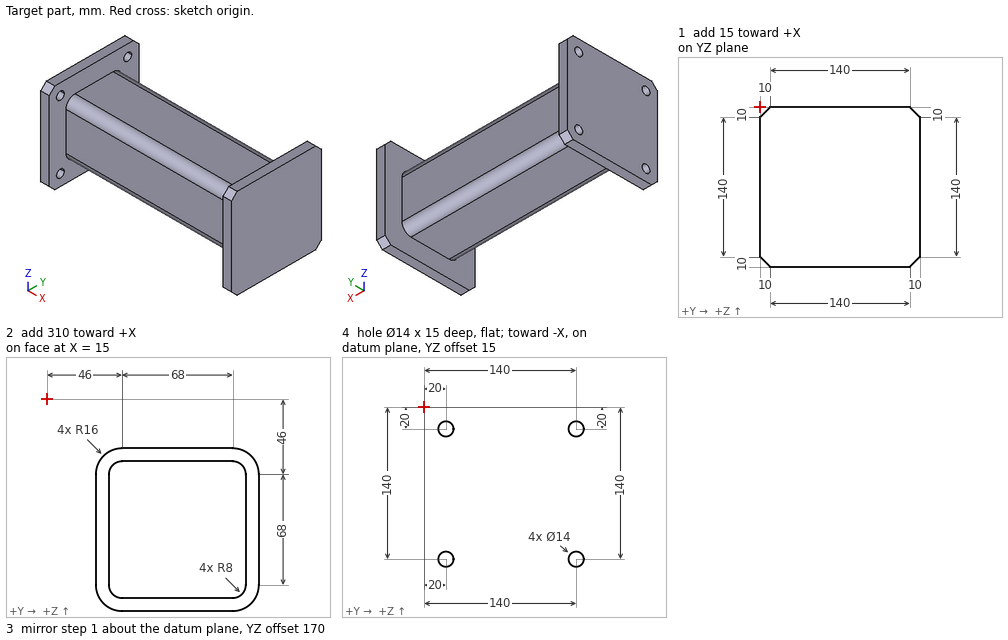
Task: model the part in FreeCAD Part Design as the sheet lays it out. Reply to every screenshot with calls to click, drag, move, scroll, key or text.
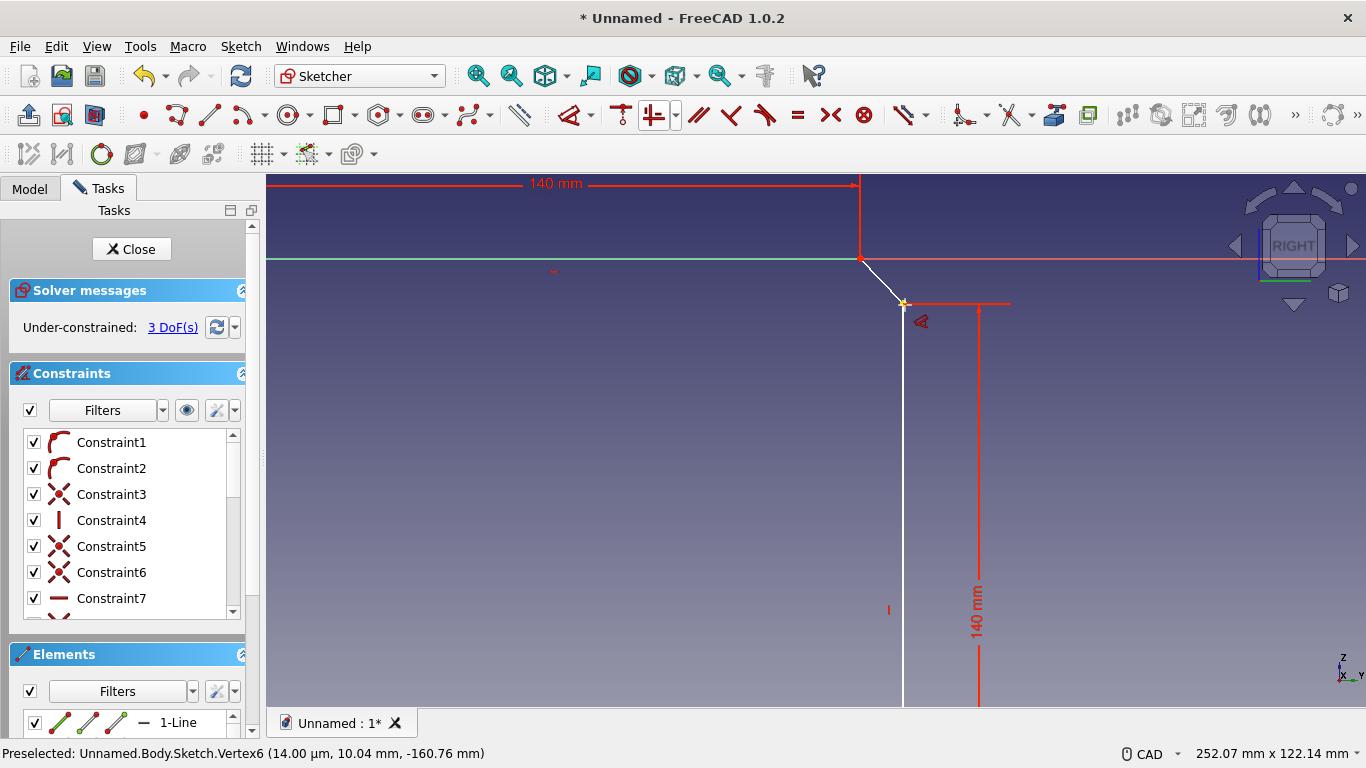
click(903, 304)
click(937, 281)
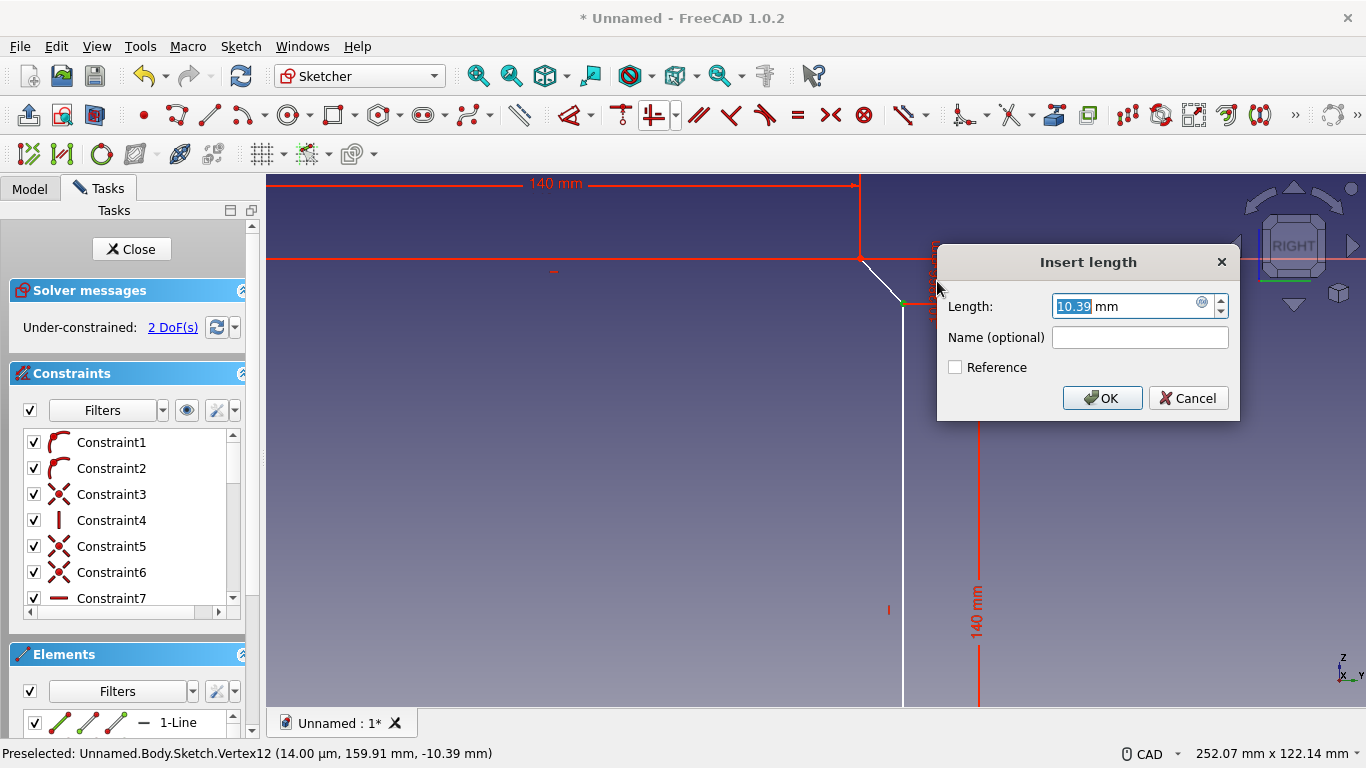
text(10)
key(Return)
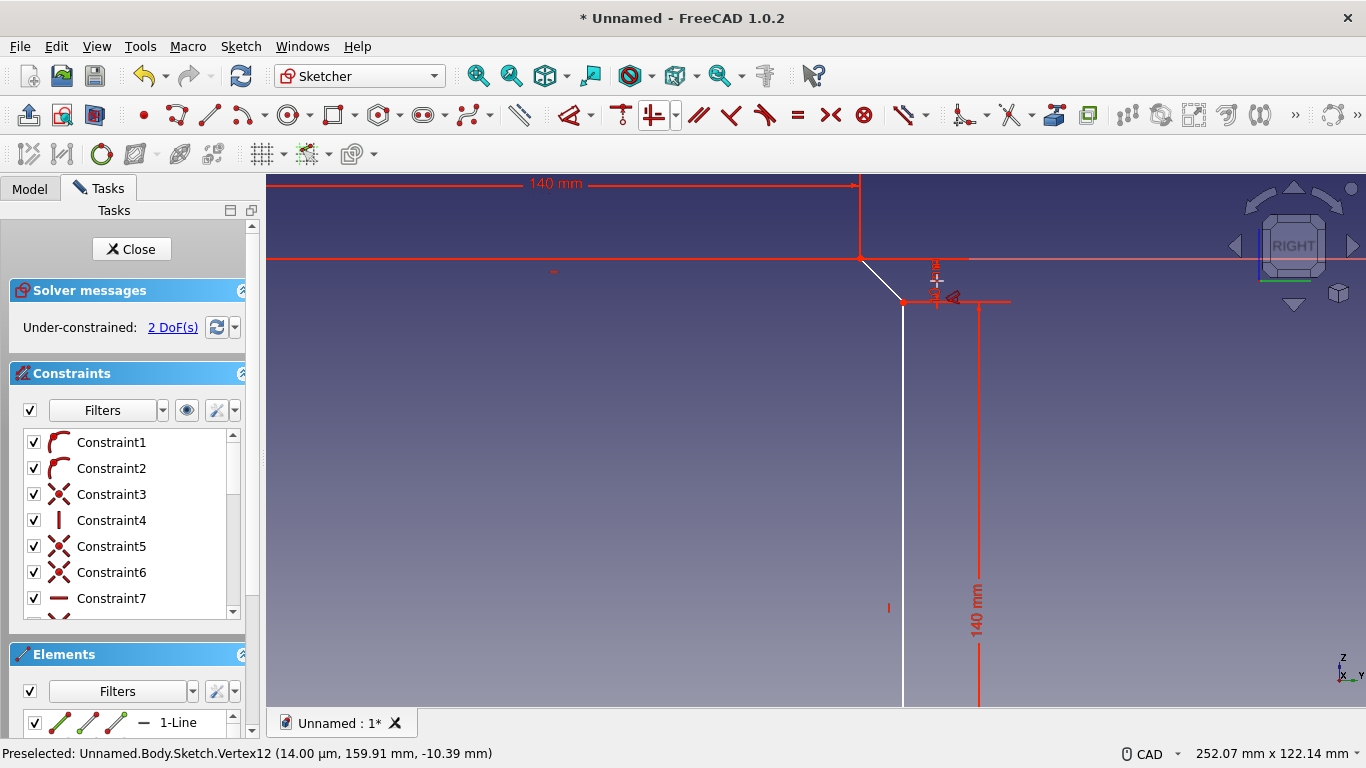
scroll(905, 304, down, 4)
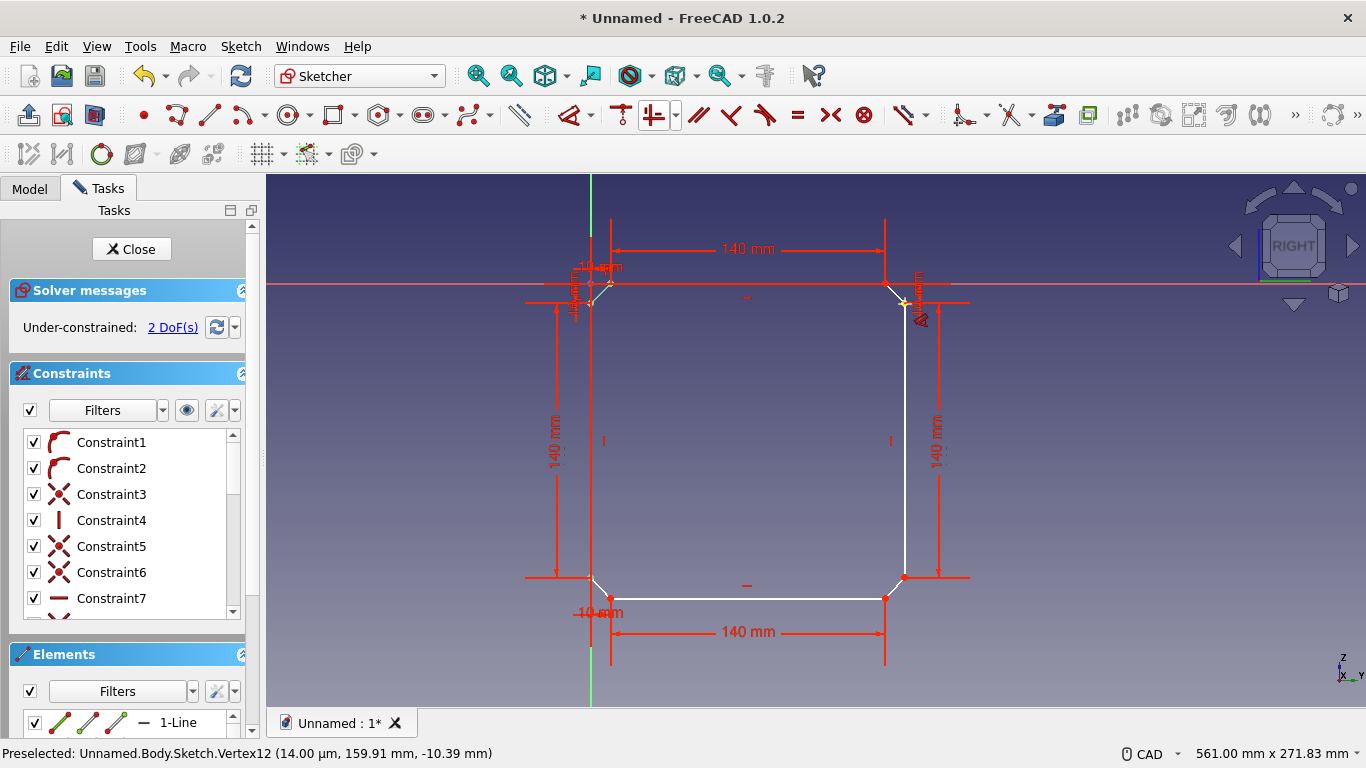
scroll(597, 584, up, 5)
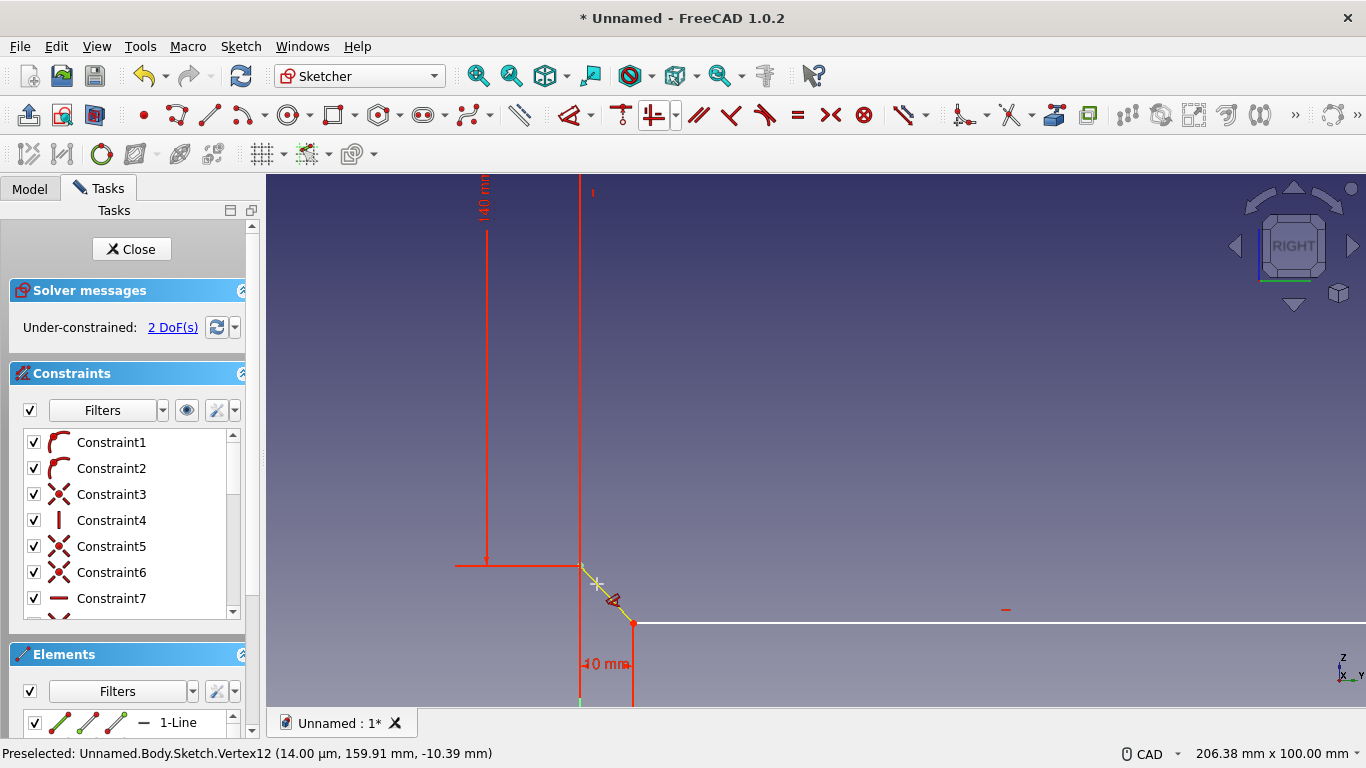
click(596, 583)
click(546, 595)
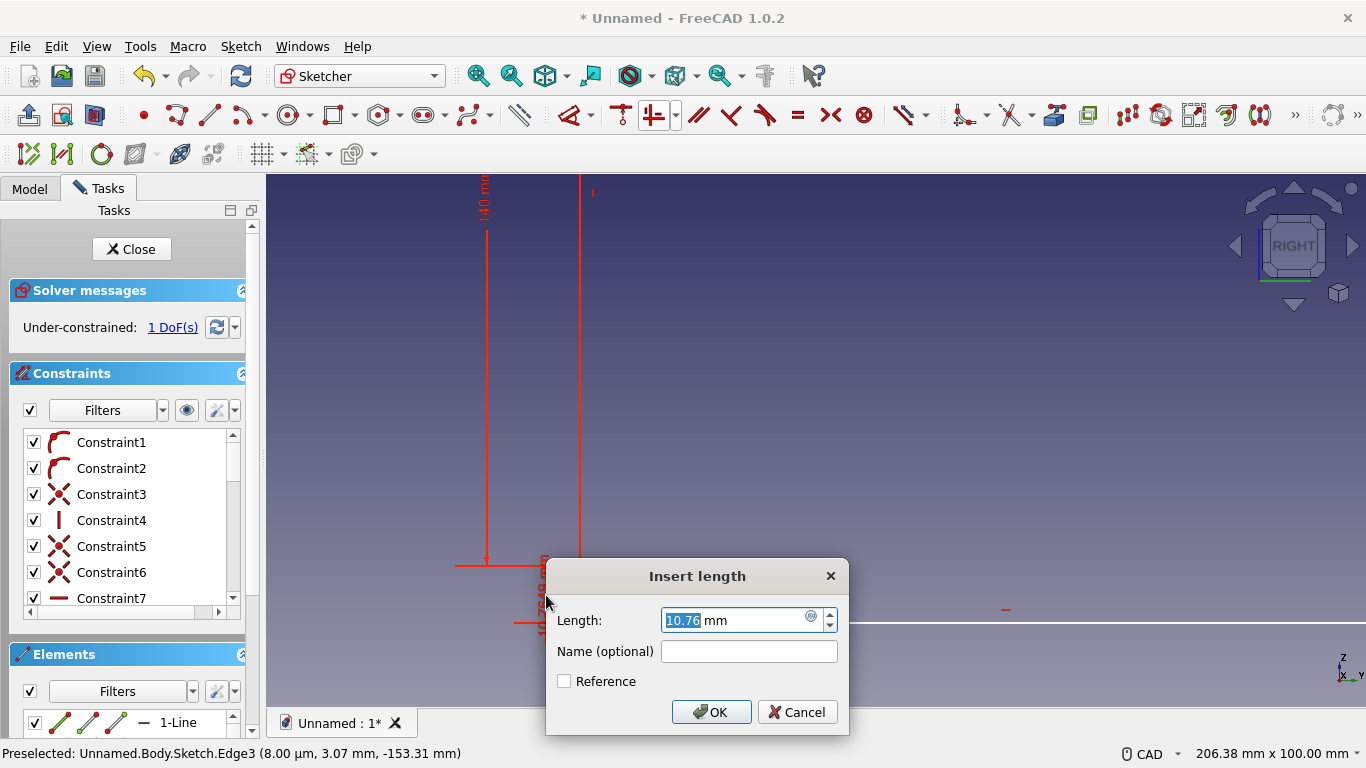
text(10)
key(Return)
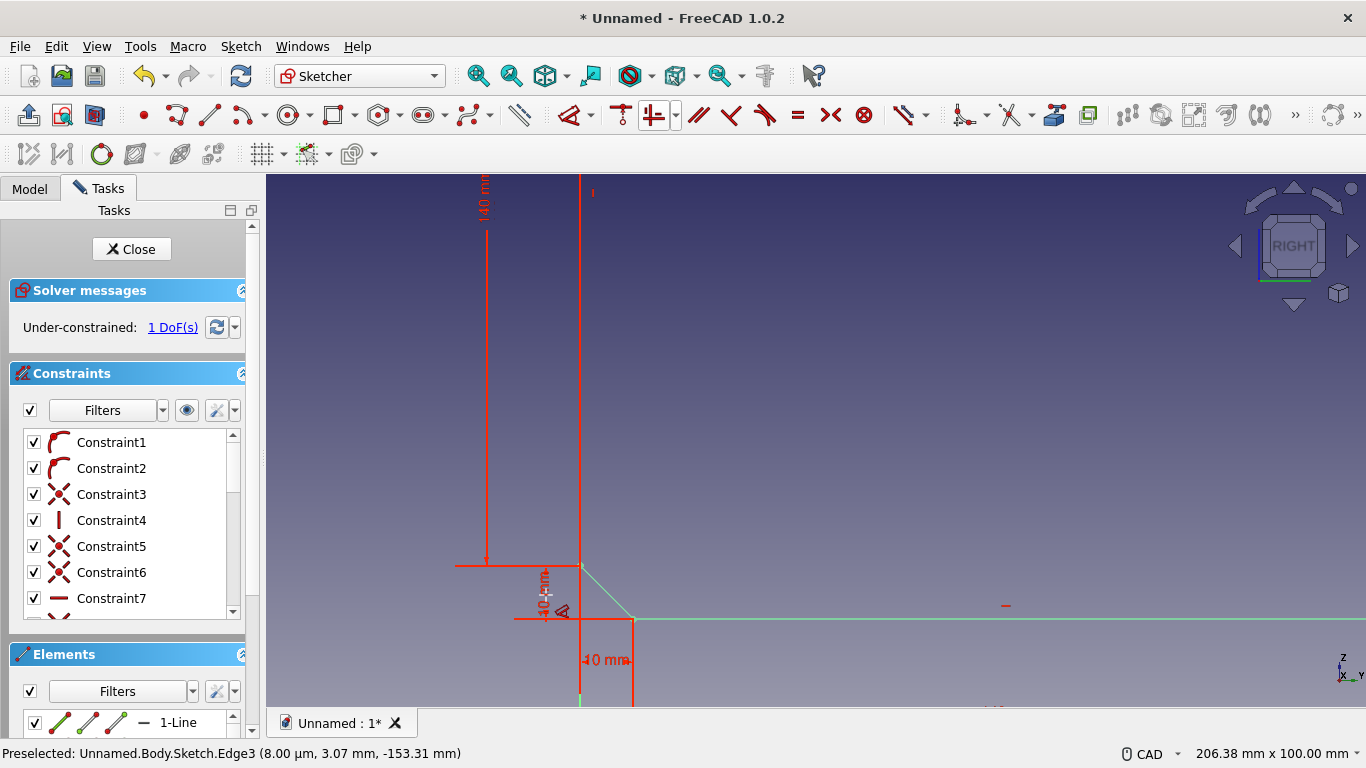
scroll(597, 585, down, 5)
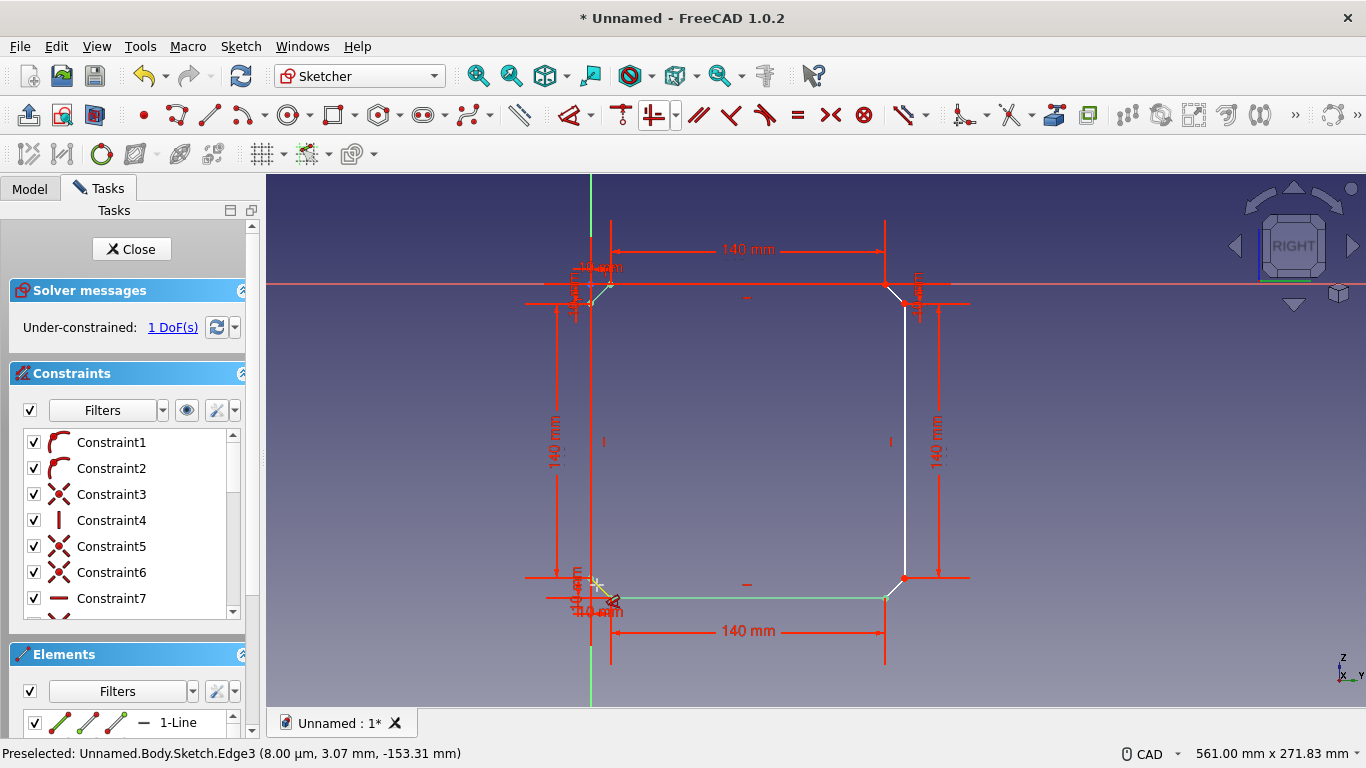
scroll(891, 592, up, 4)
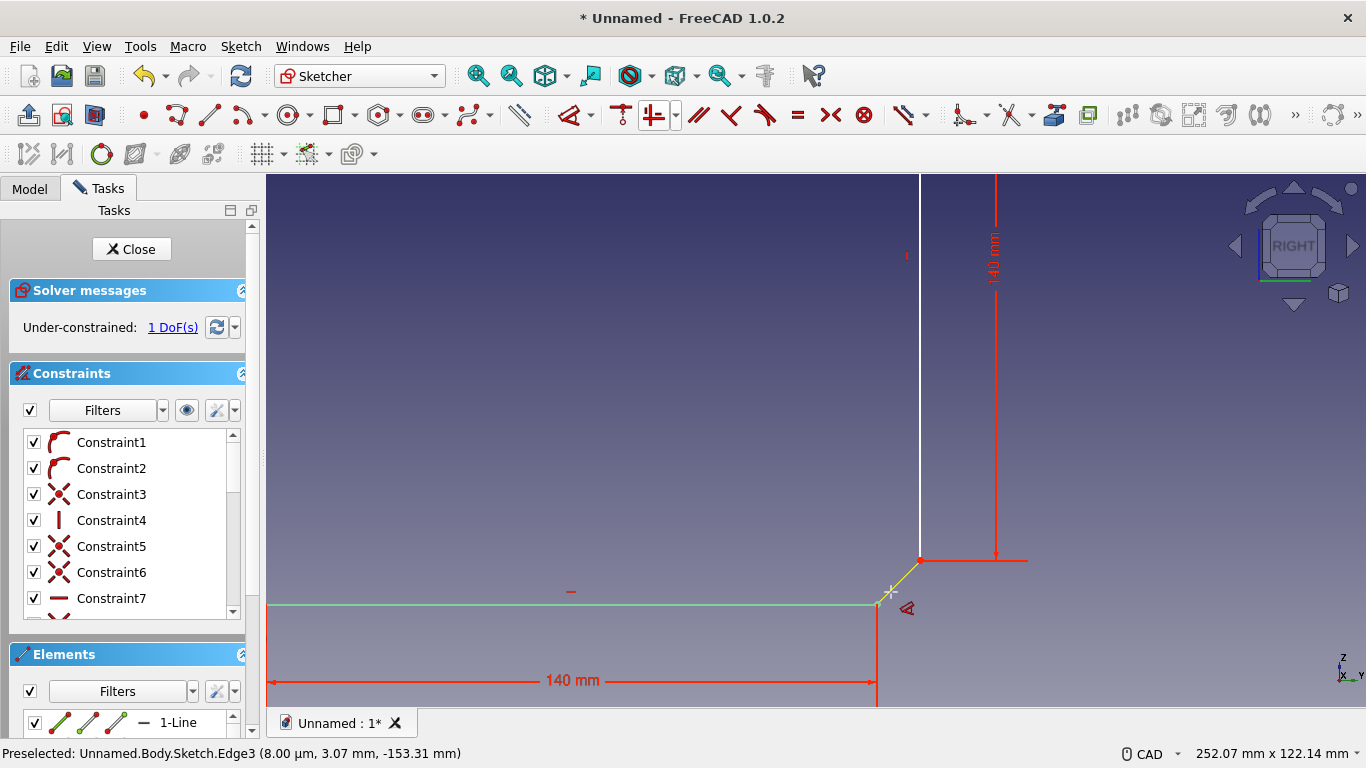
click(890, 591)
click(899, 639)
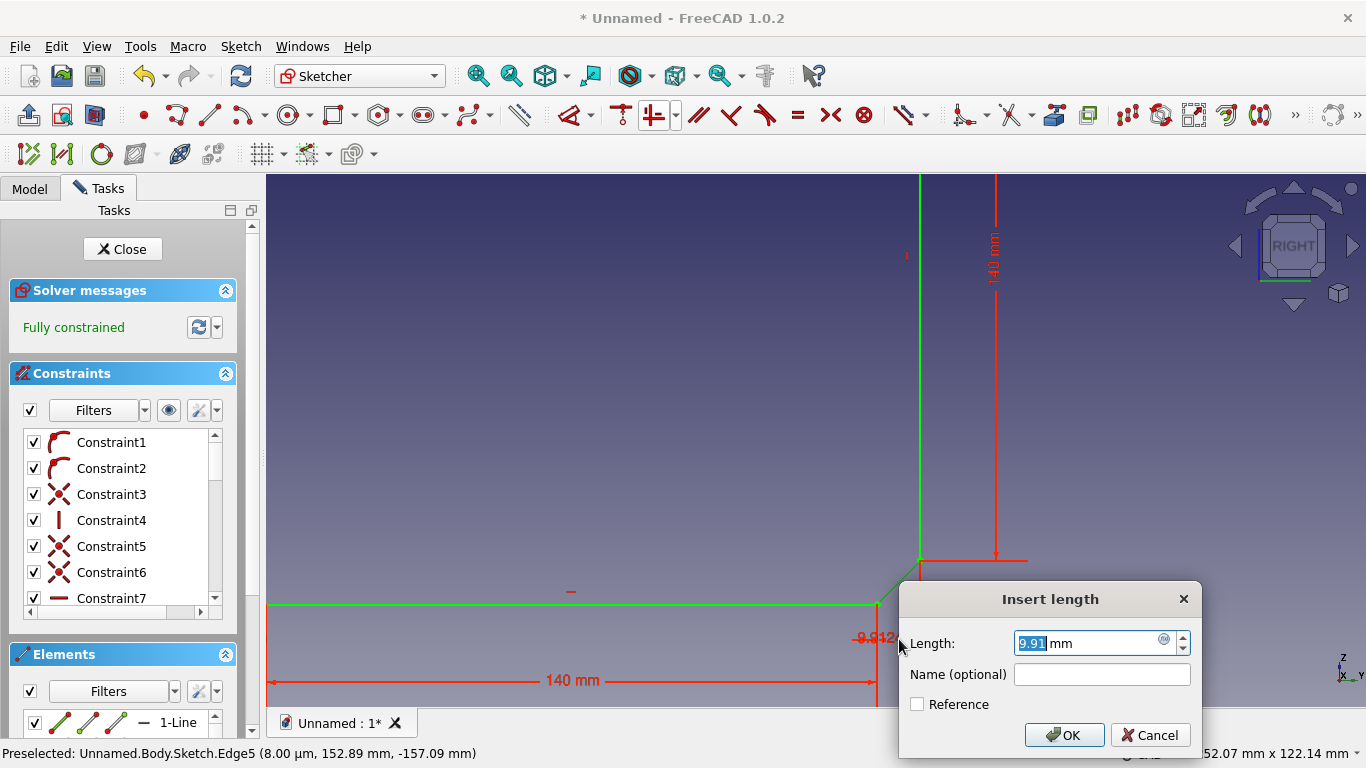
text(10)
key(Return)
key(Escape)